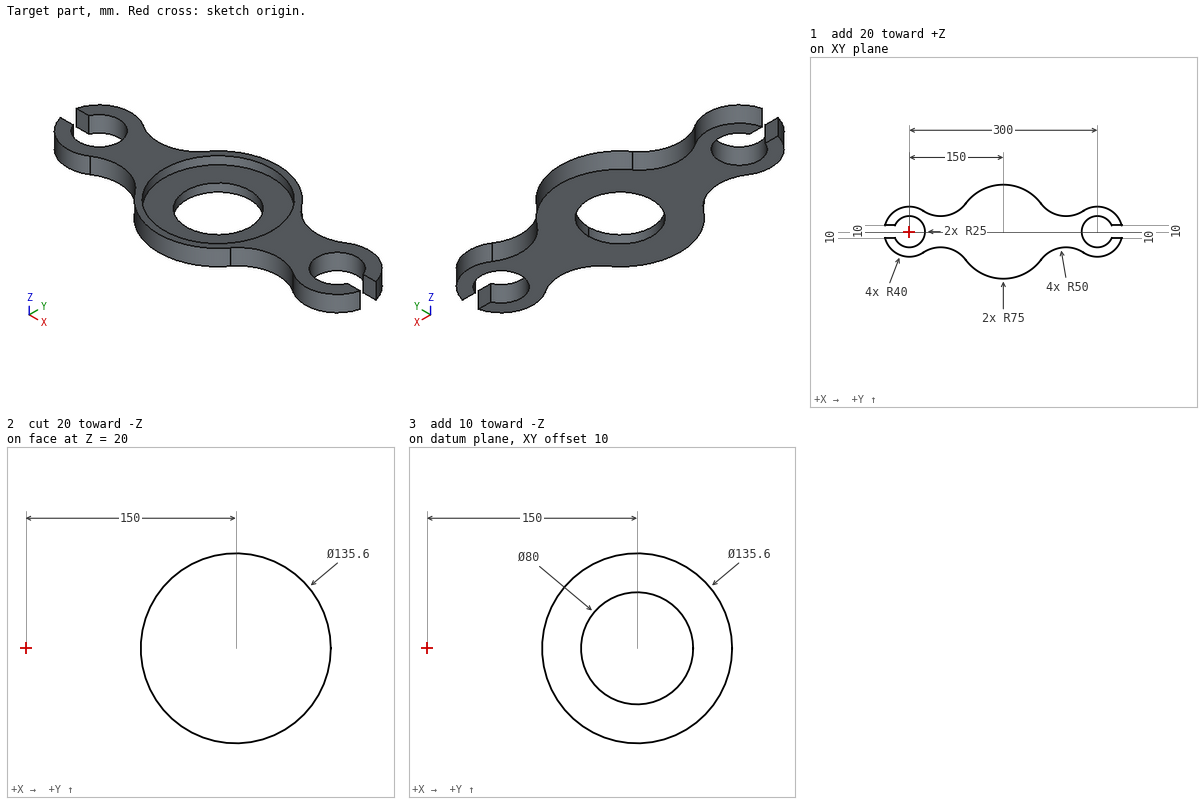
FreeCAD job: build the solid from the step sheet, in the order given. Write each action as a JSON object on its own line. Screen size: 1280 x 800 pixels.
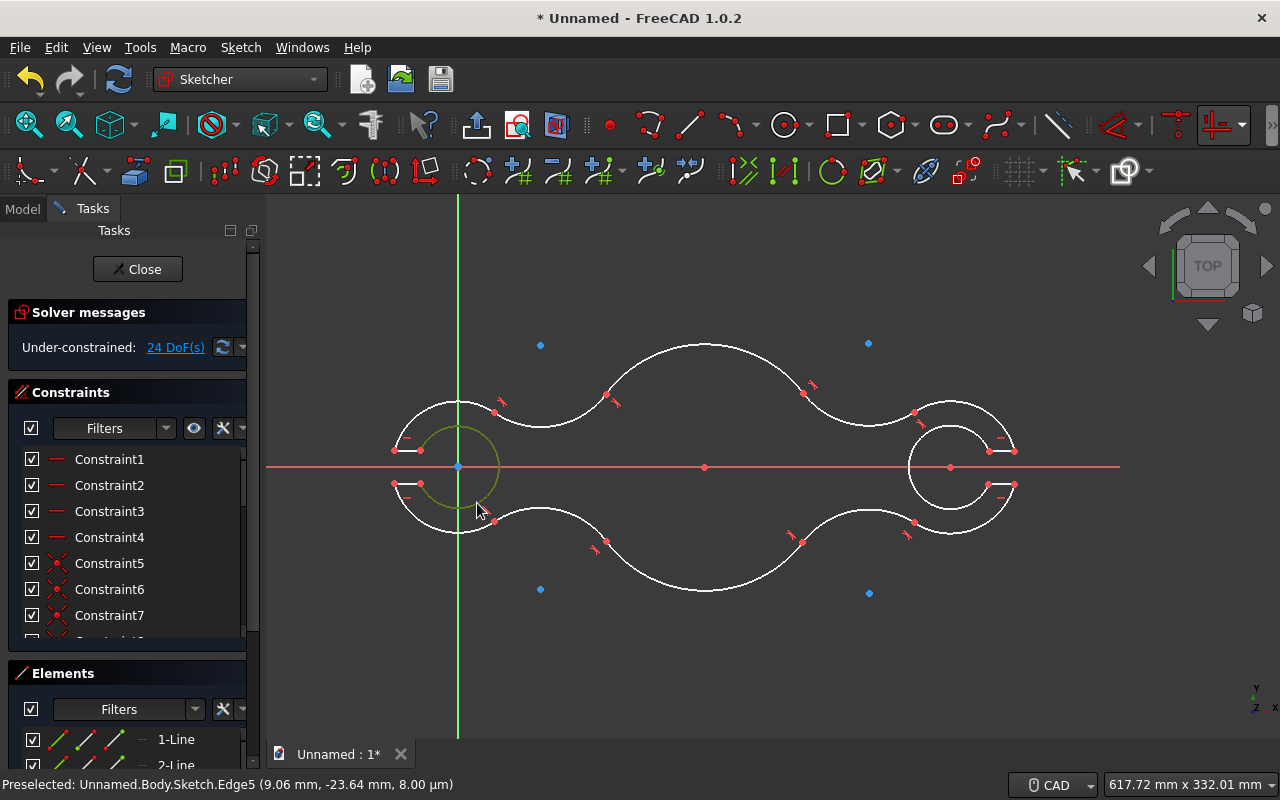
{"action": "left_click", "coordinate": [459, 401]}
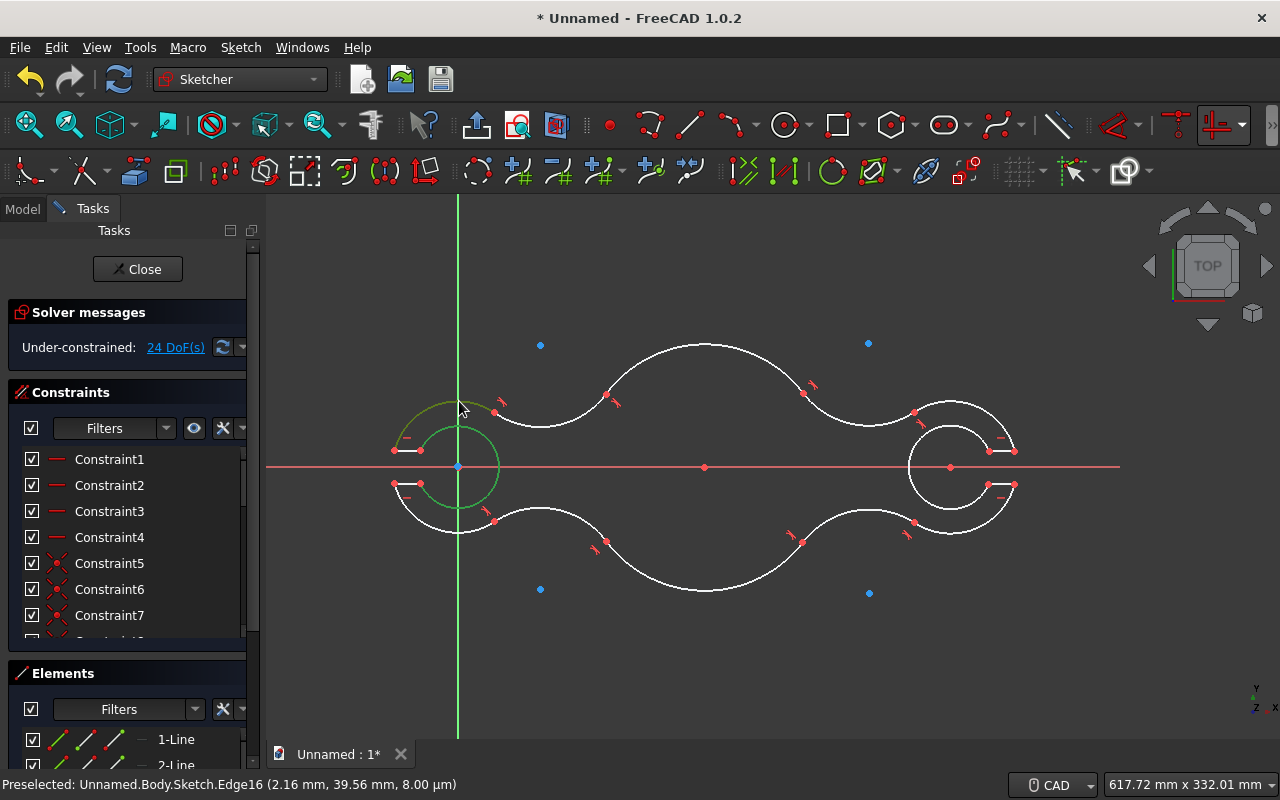
{"action": "left_click", "coordinate": [1176, 126]}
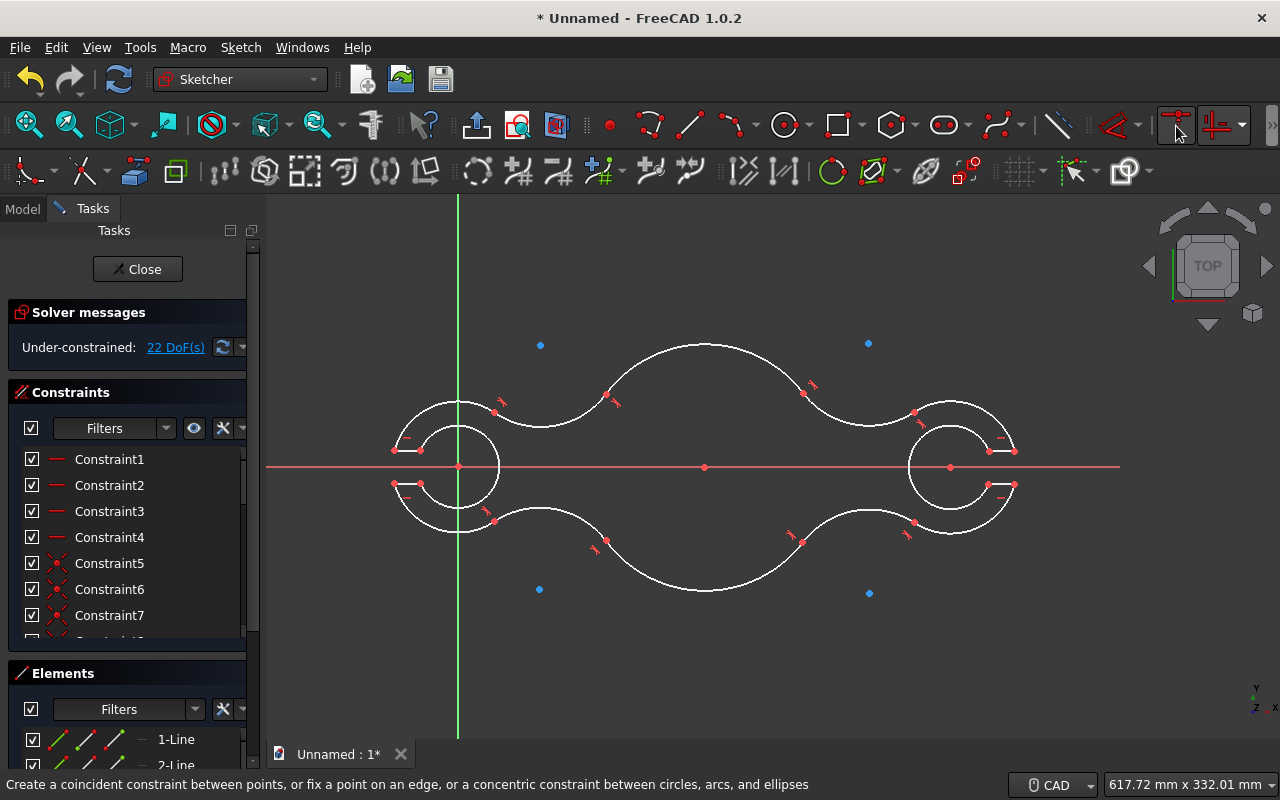
{"action": "left_click_drag", "start_coordinate": [448, 456], "coordinate": [468, 477]}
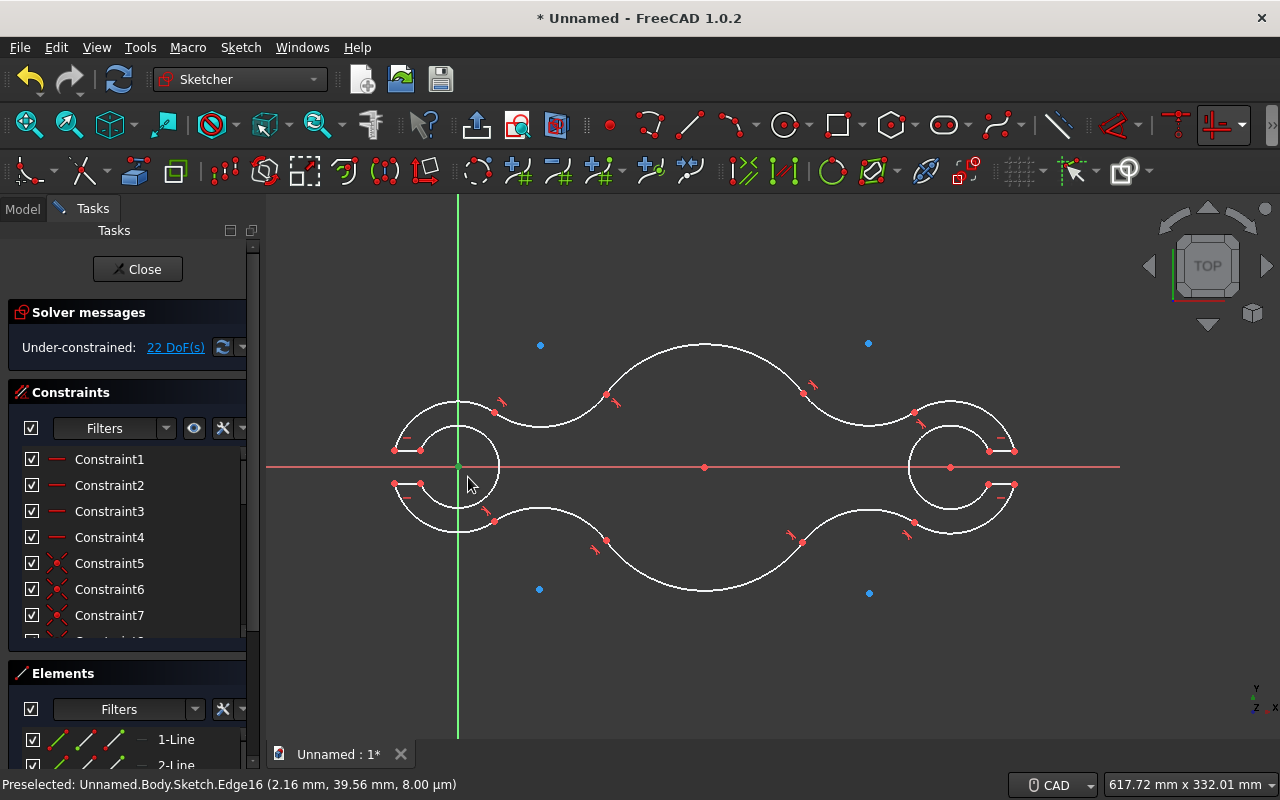
{"action": "left_click", "coordinate": [1176, 126]}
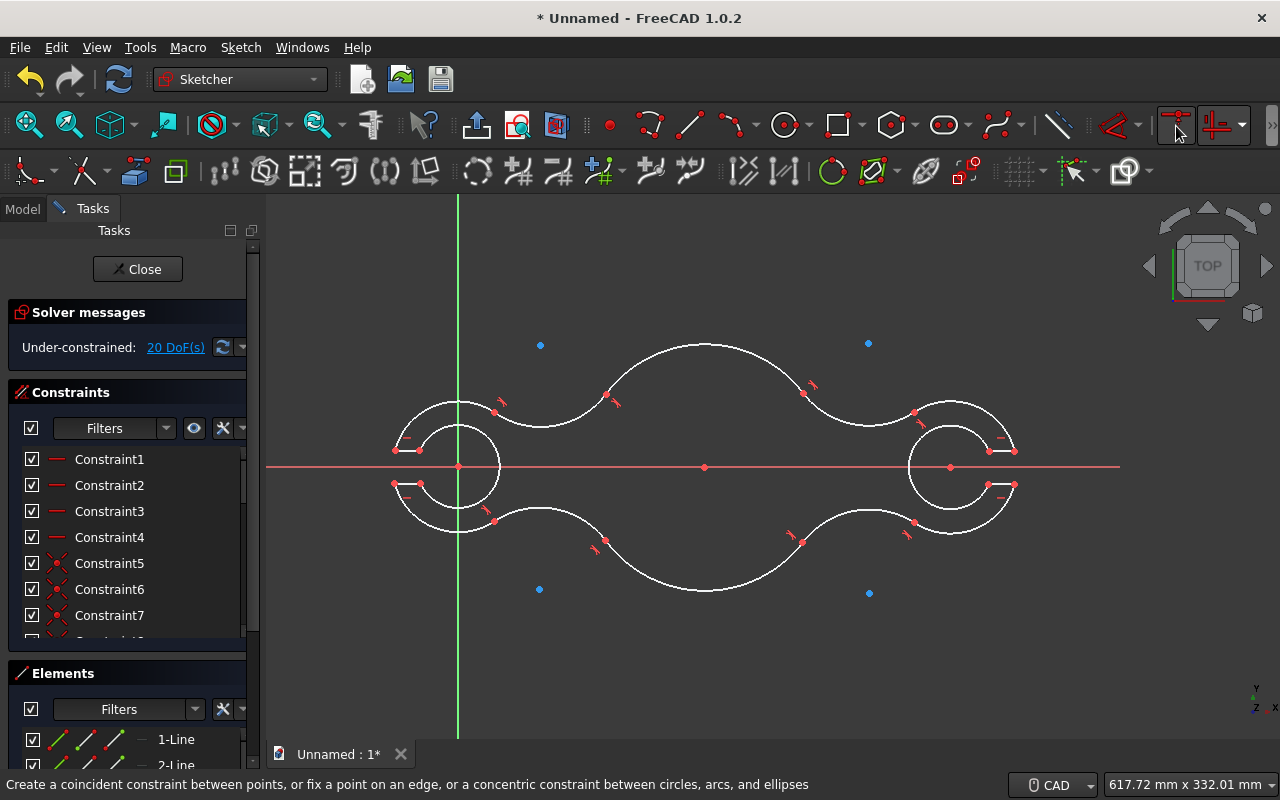
{"action": "left_click", "coordinate": [578, 517]}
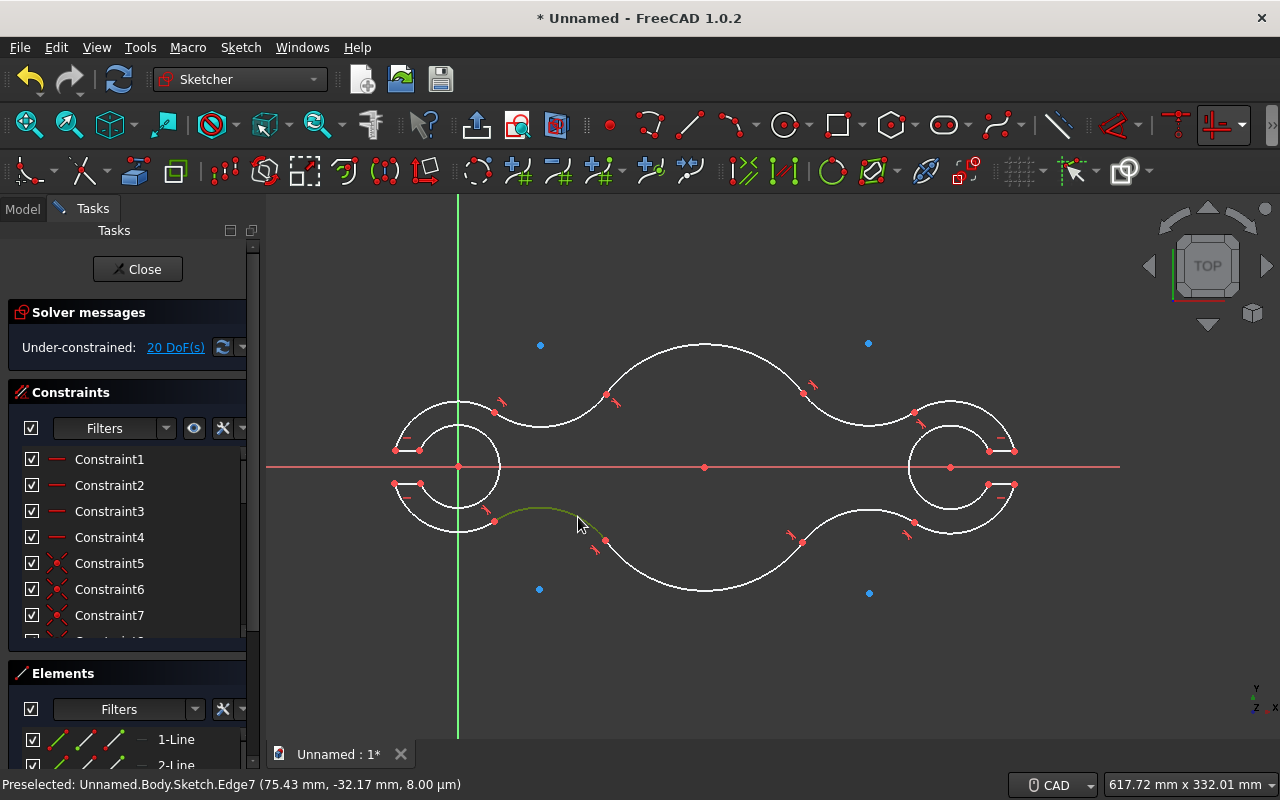
{"action": "left_click", "coordinate": [880, 510]}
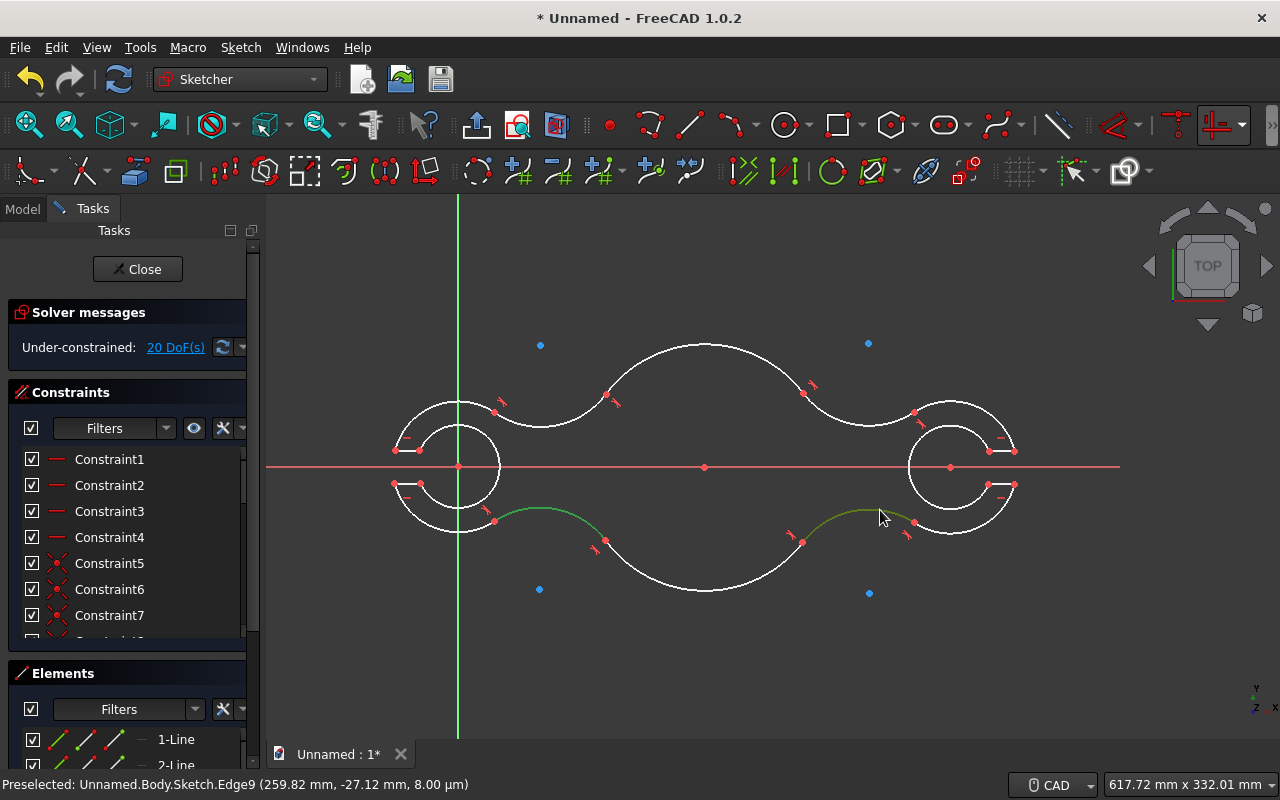
{"action": "left_click", "coordinate": [831, 417]}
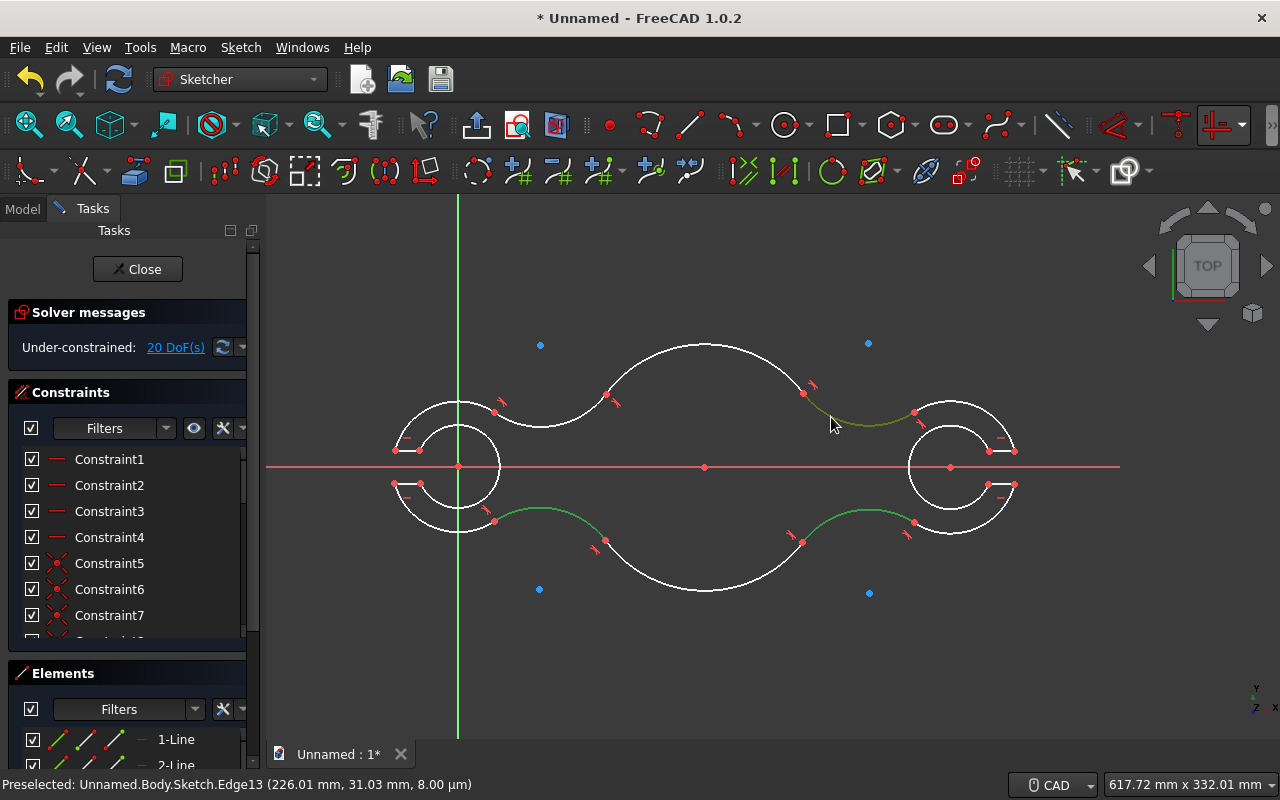
{"action": "left_click", "coordinate": [529, 426]}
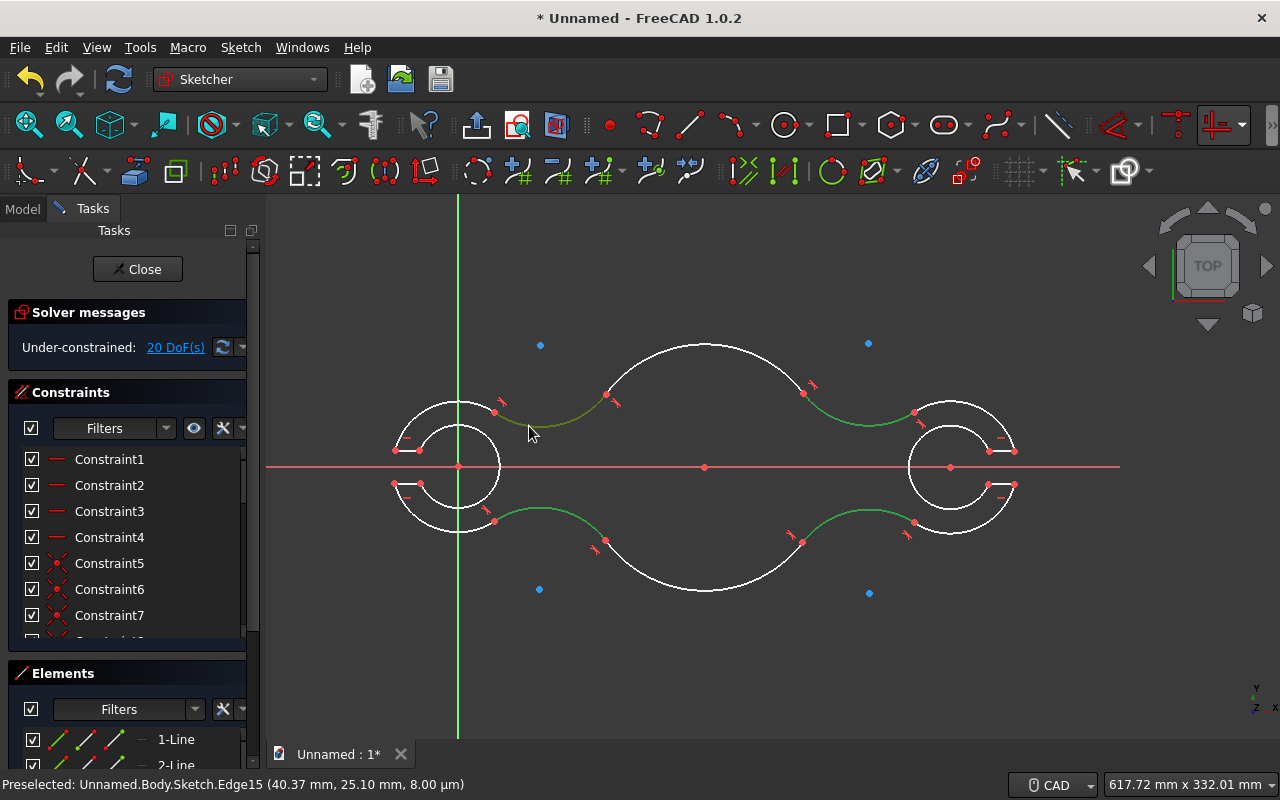
{"action": "key", "text": "e"}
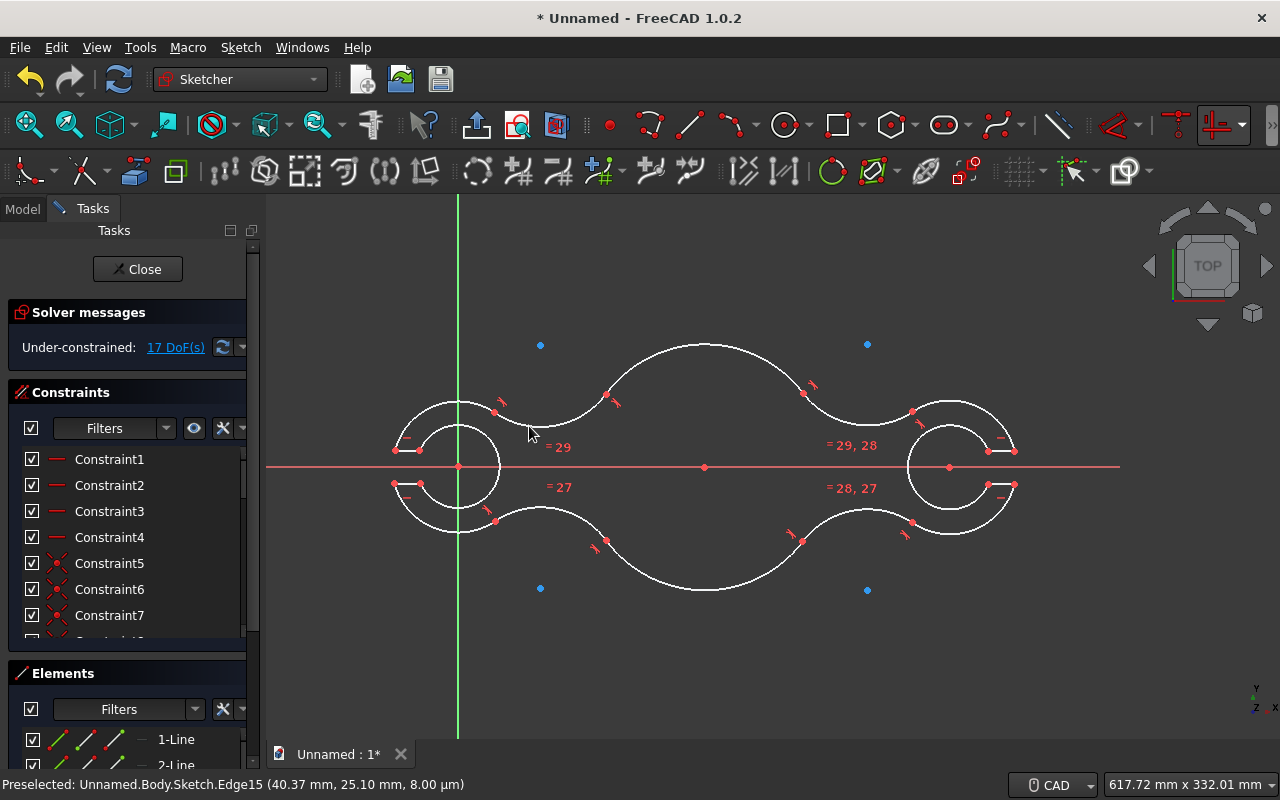
{"action": "left_click", "coordinate": [414, 516]}